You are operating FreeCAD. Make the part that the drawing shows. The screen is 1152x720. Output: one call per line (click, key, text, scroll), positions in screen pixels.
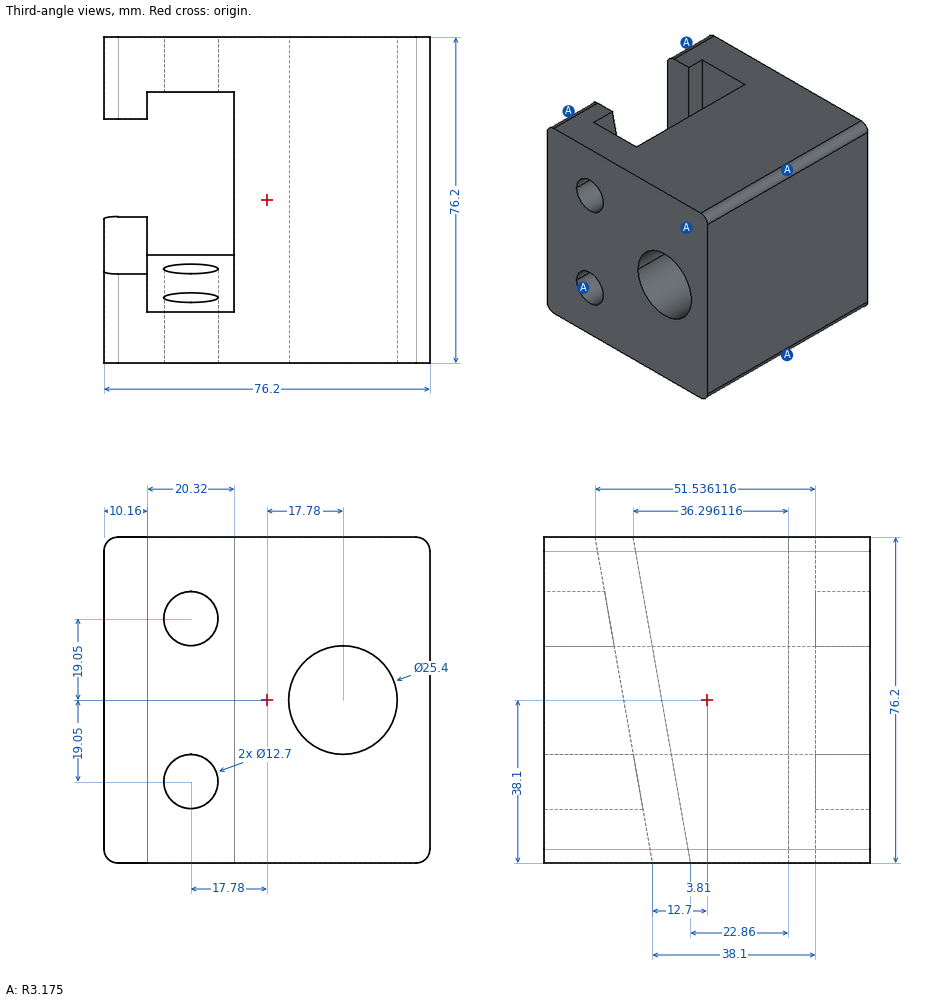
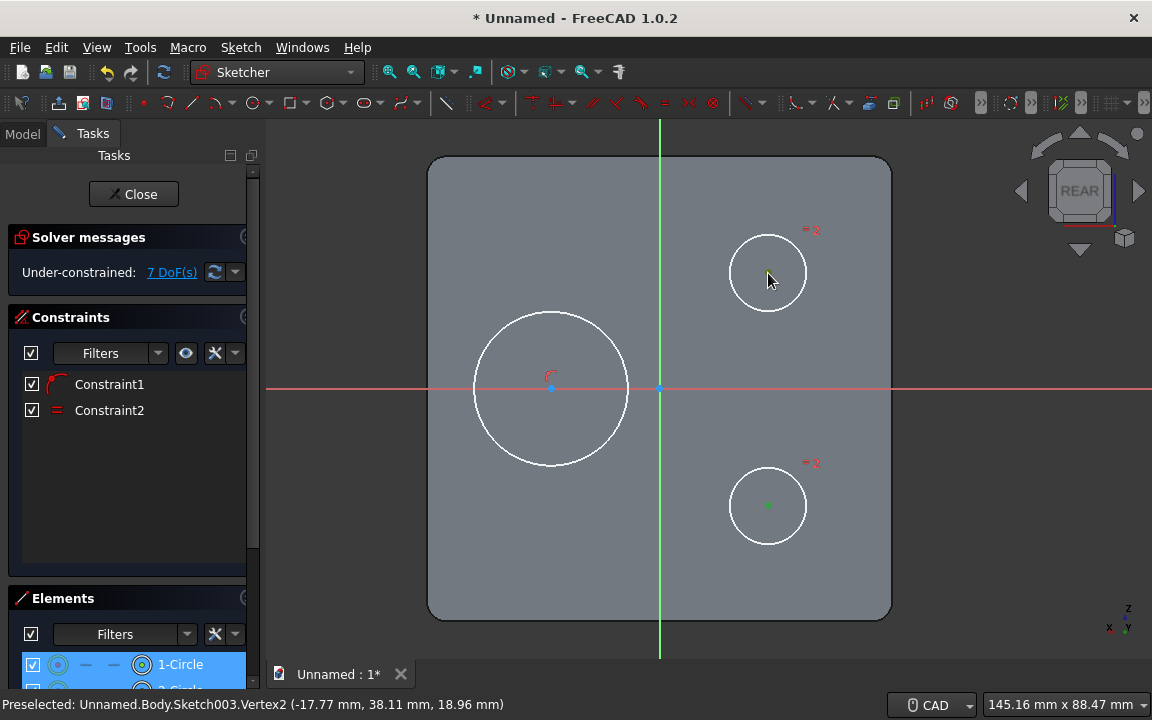
key(v)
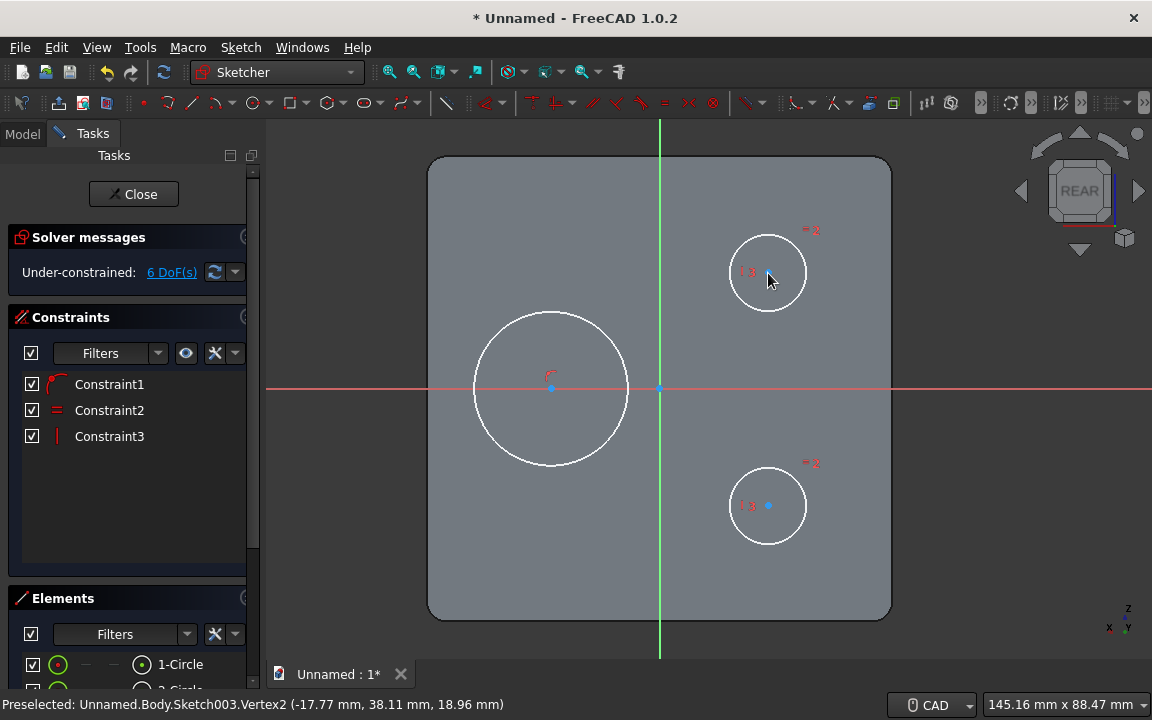
click(486, 104)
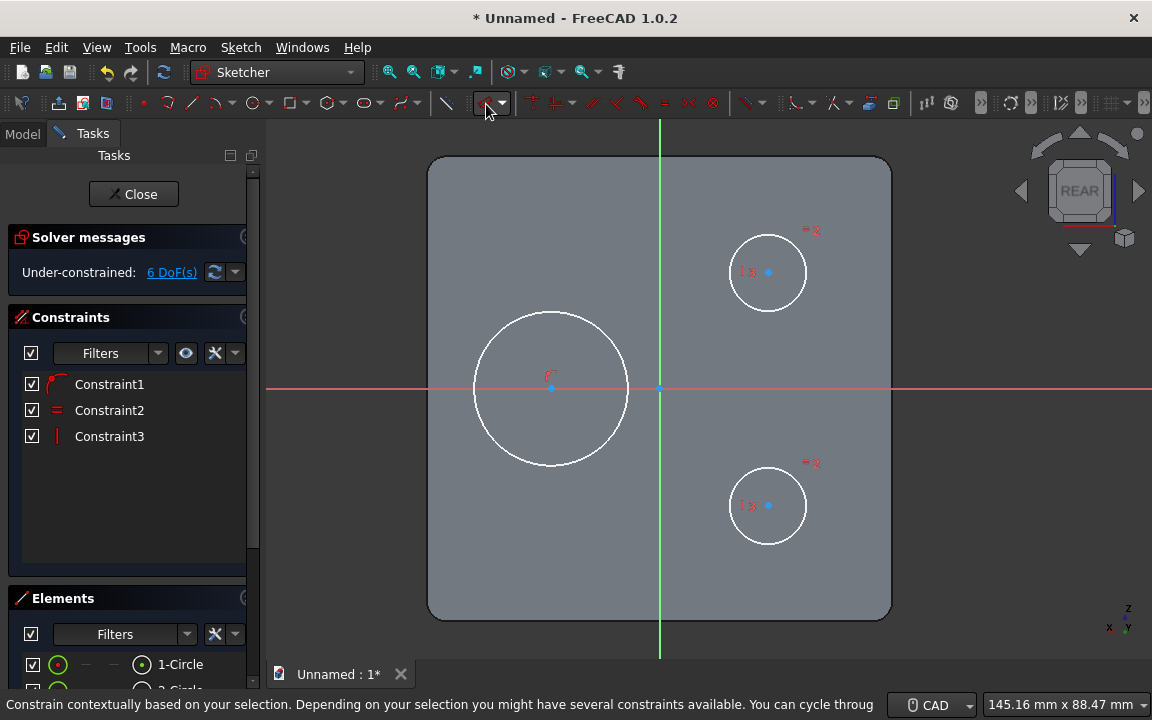
click(795, 479)
click(818, 456)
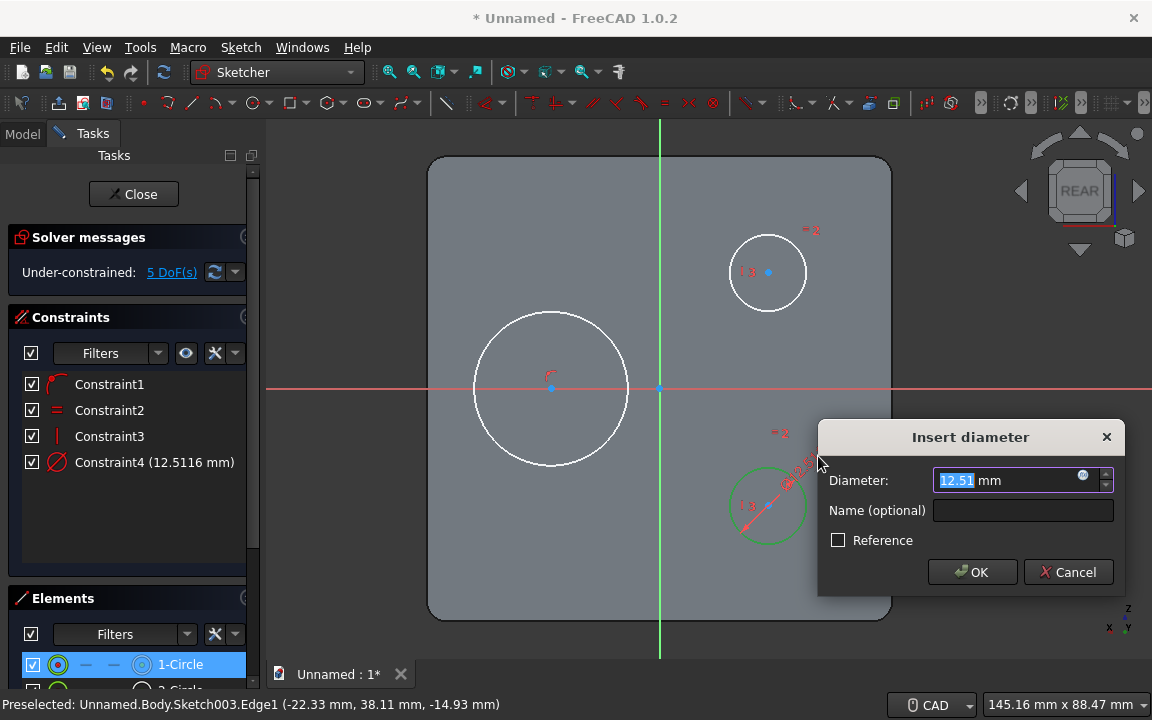
text(12.7)
key(Return)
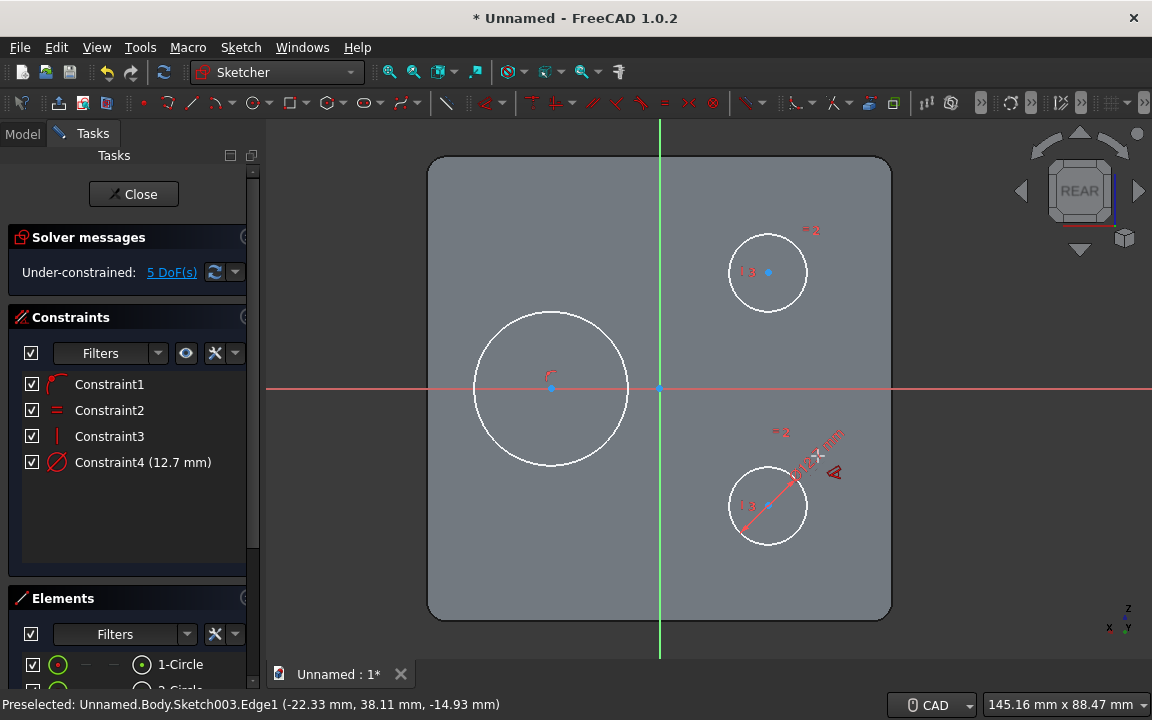
click(605, 334)
click(627, 311)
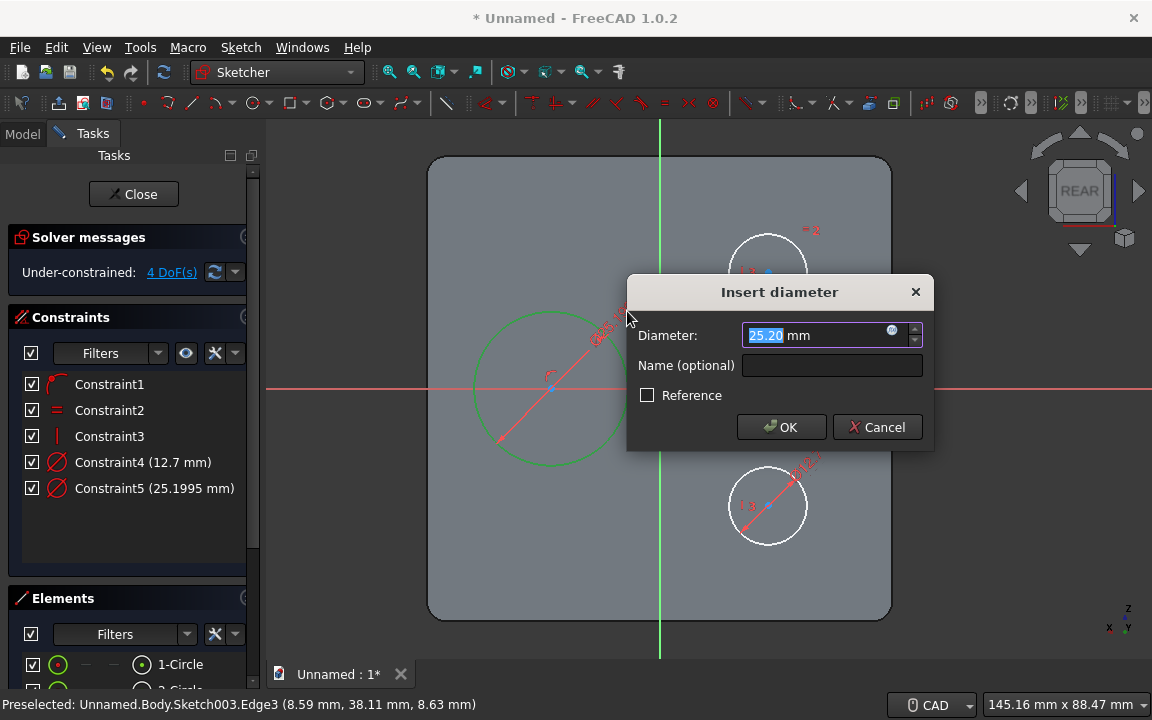
text(25.4)
key(Return)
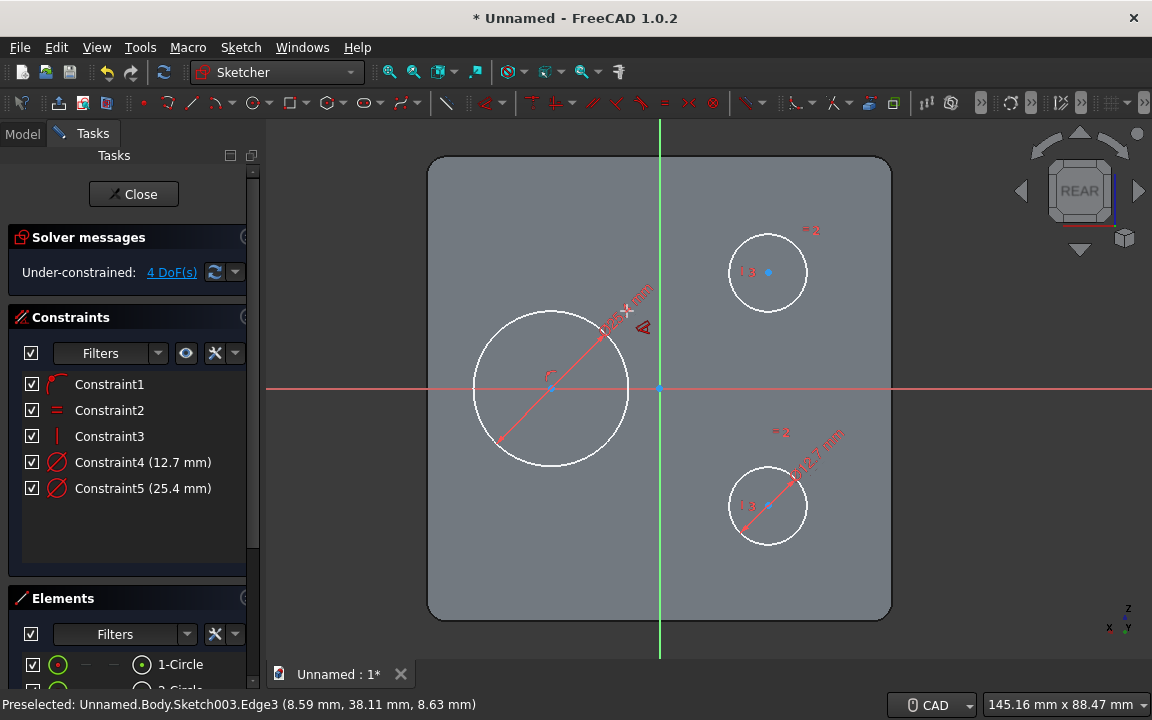
click(768, 506)
click(714, 540)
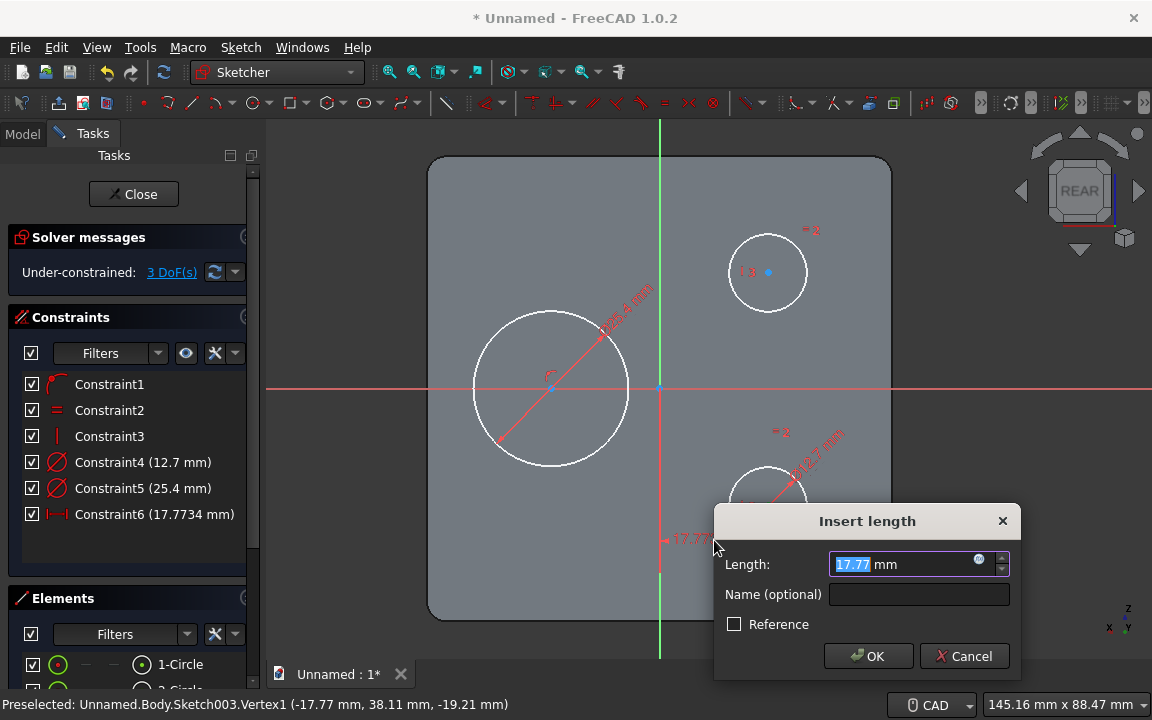
text(17.78)
key(Return)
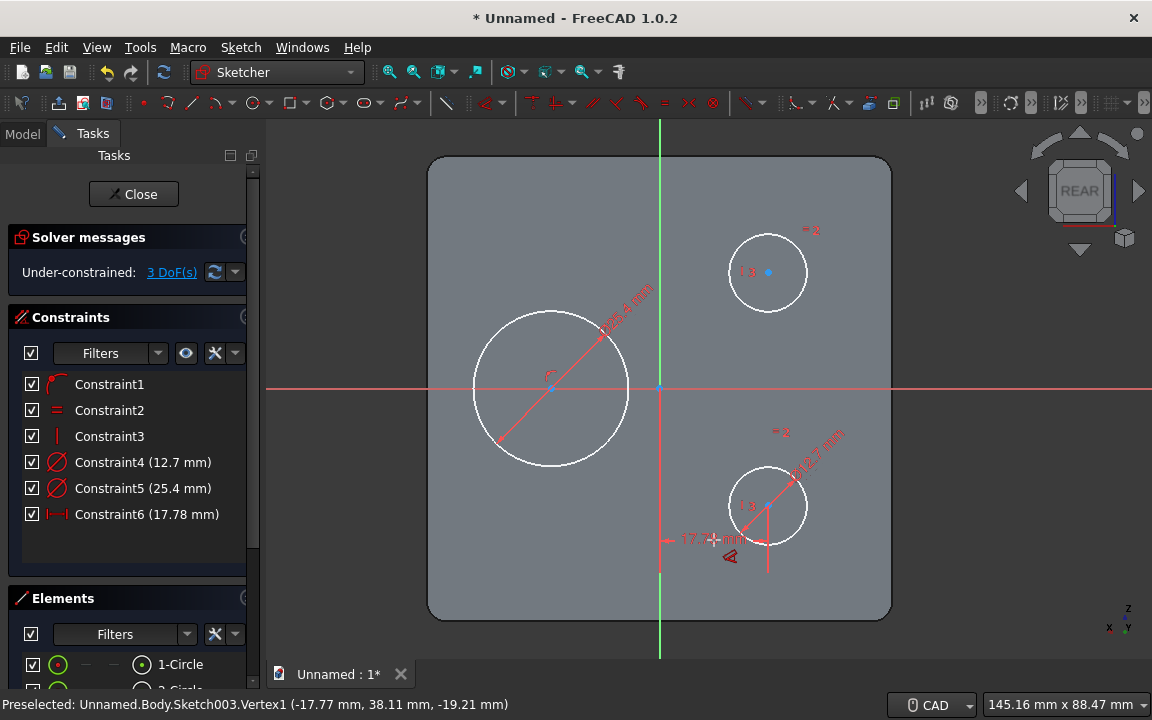
click(768, 506)
click(802, 420)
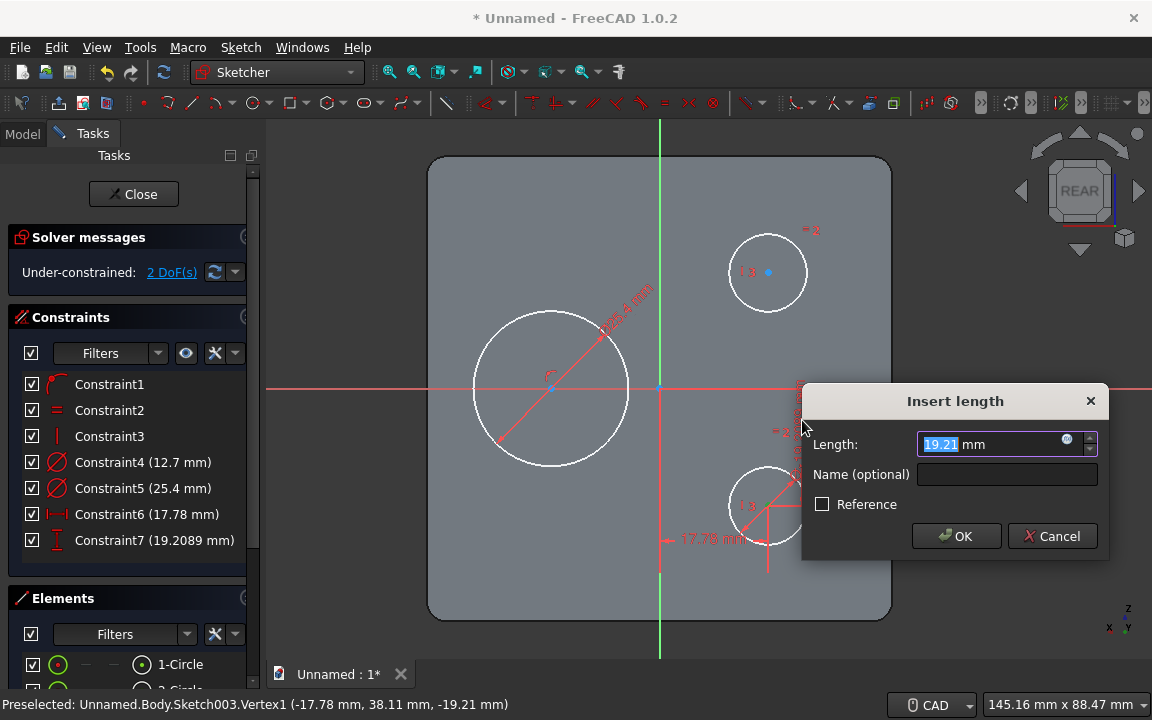
text(19.05)
key(Return)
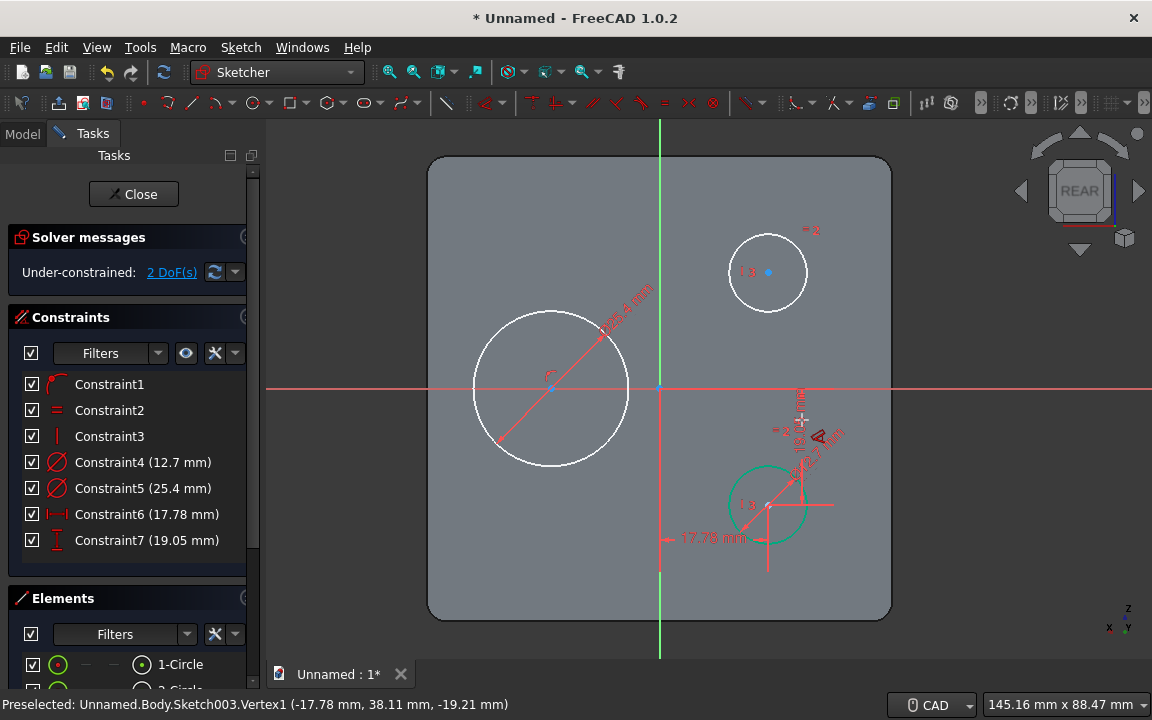
click(768, 273)
click(802, 331)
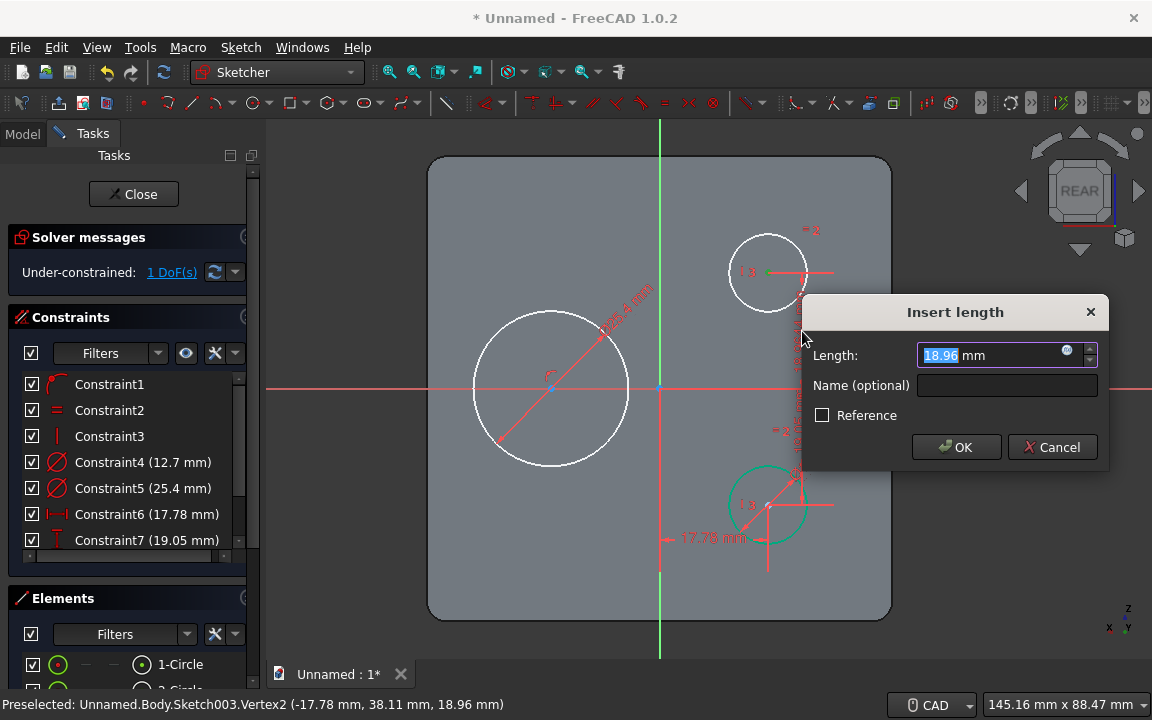
text(19.05)
key(Return)